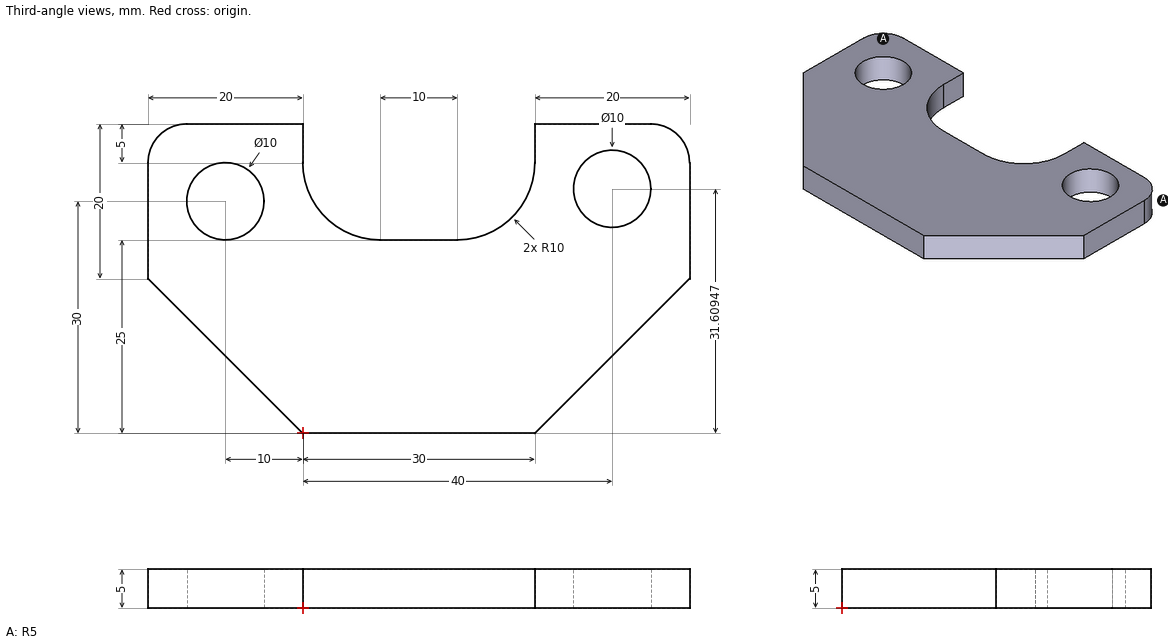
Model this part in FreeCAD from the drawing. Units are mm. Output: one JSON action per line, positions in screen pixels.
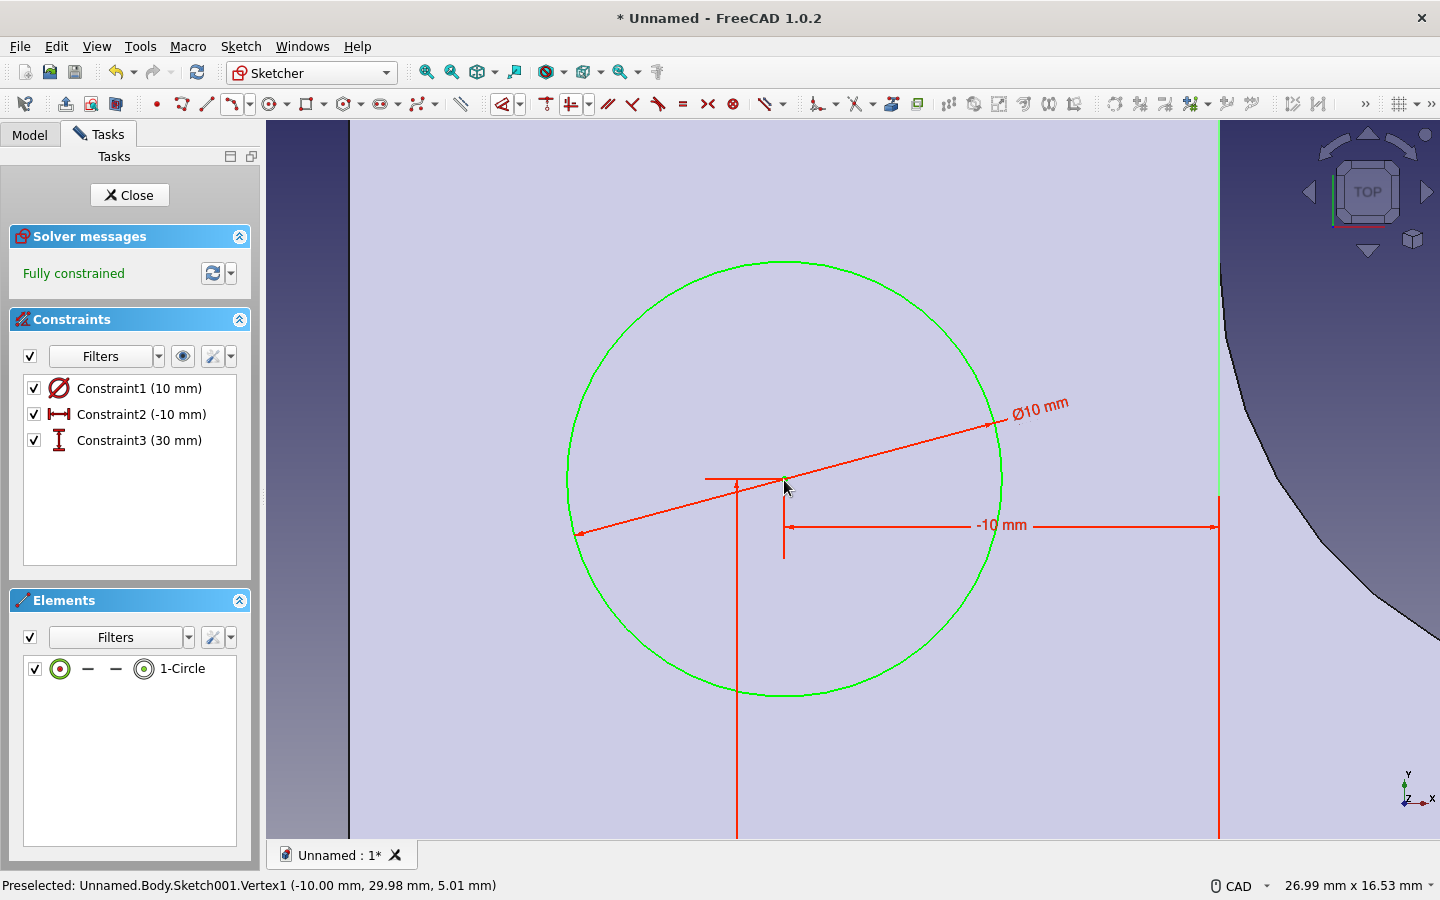
{"action": "left_click", "coordinate": [130, 195]}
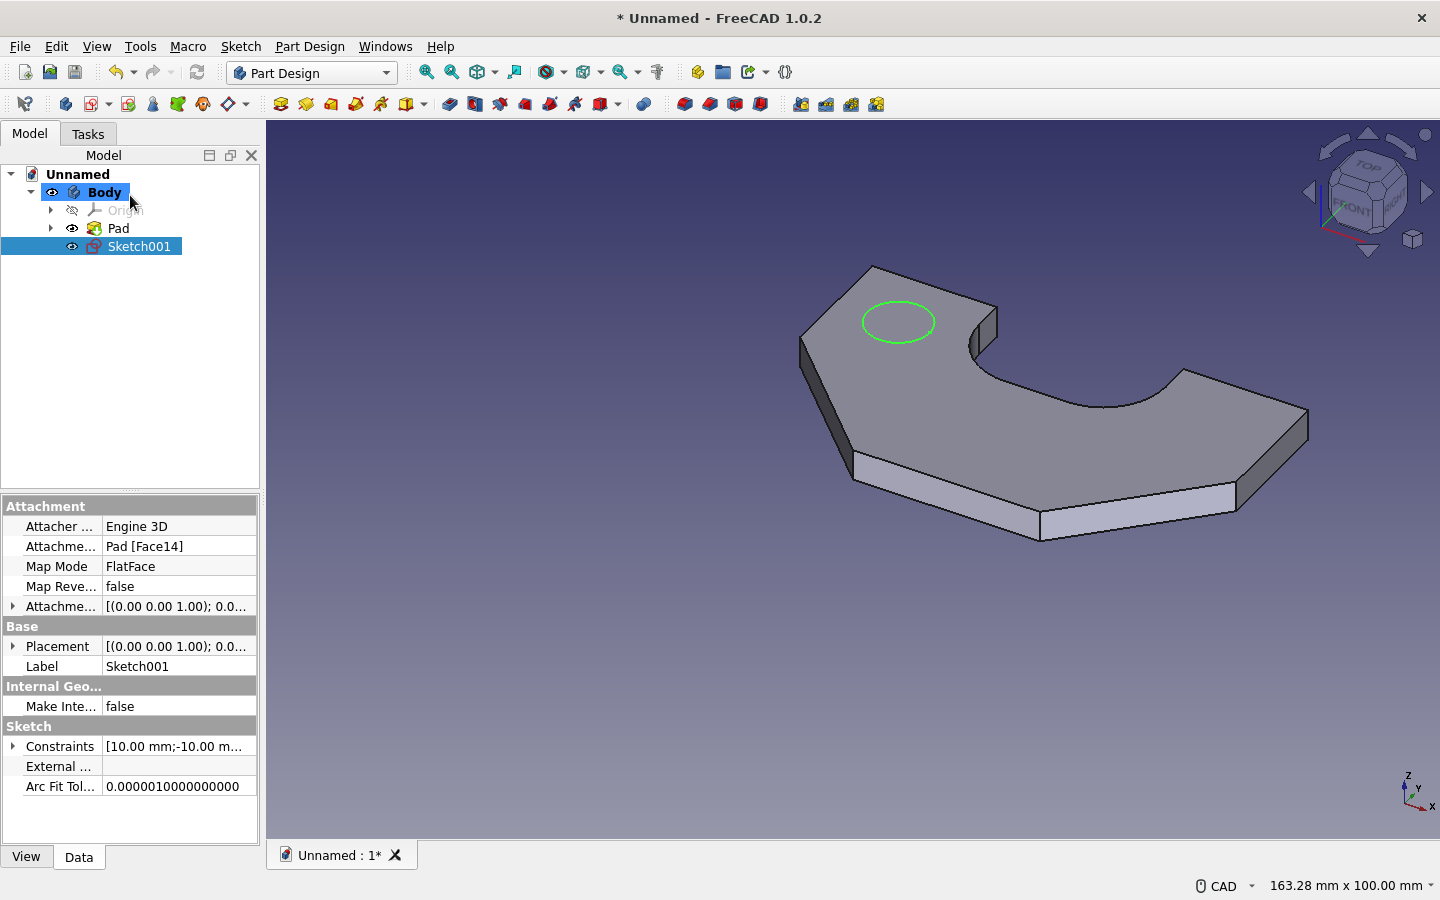
{"action": "left_click", "coordinate": [450, 104]}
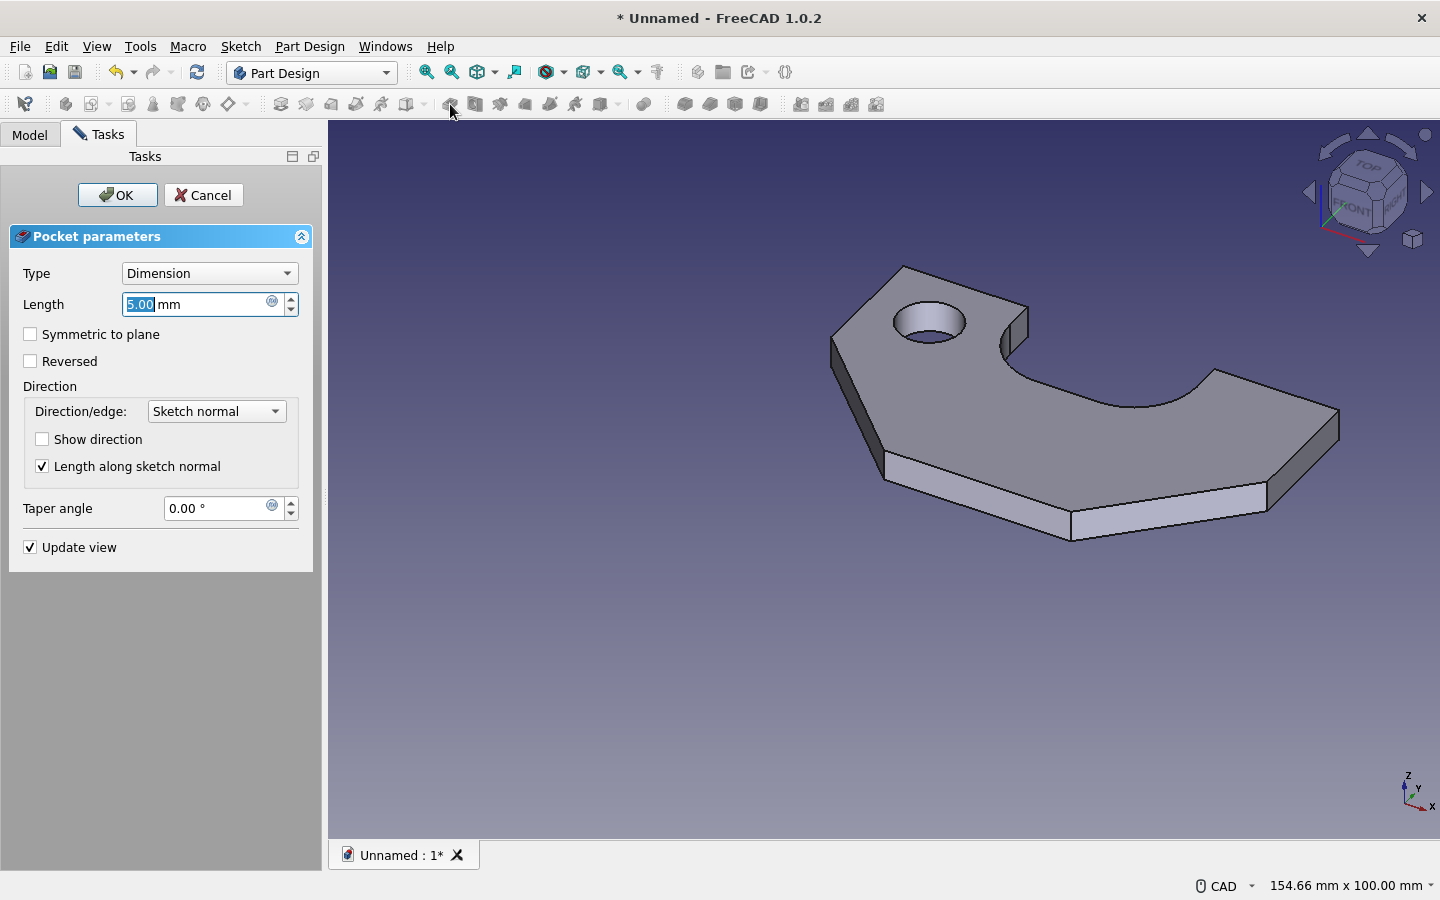
{"action": "type", "text": "5"}
{"action": "key", "text": "Tab"}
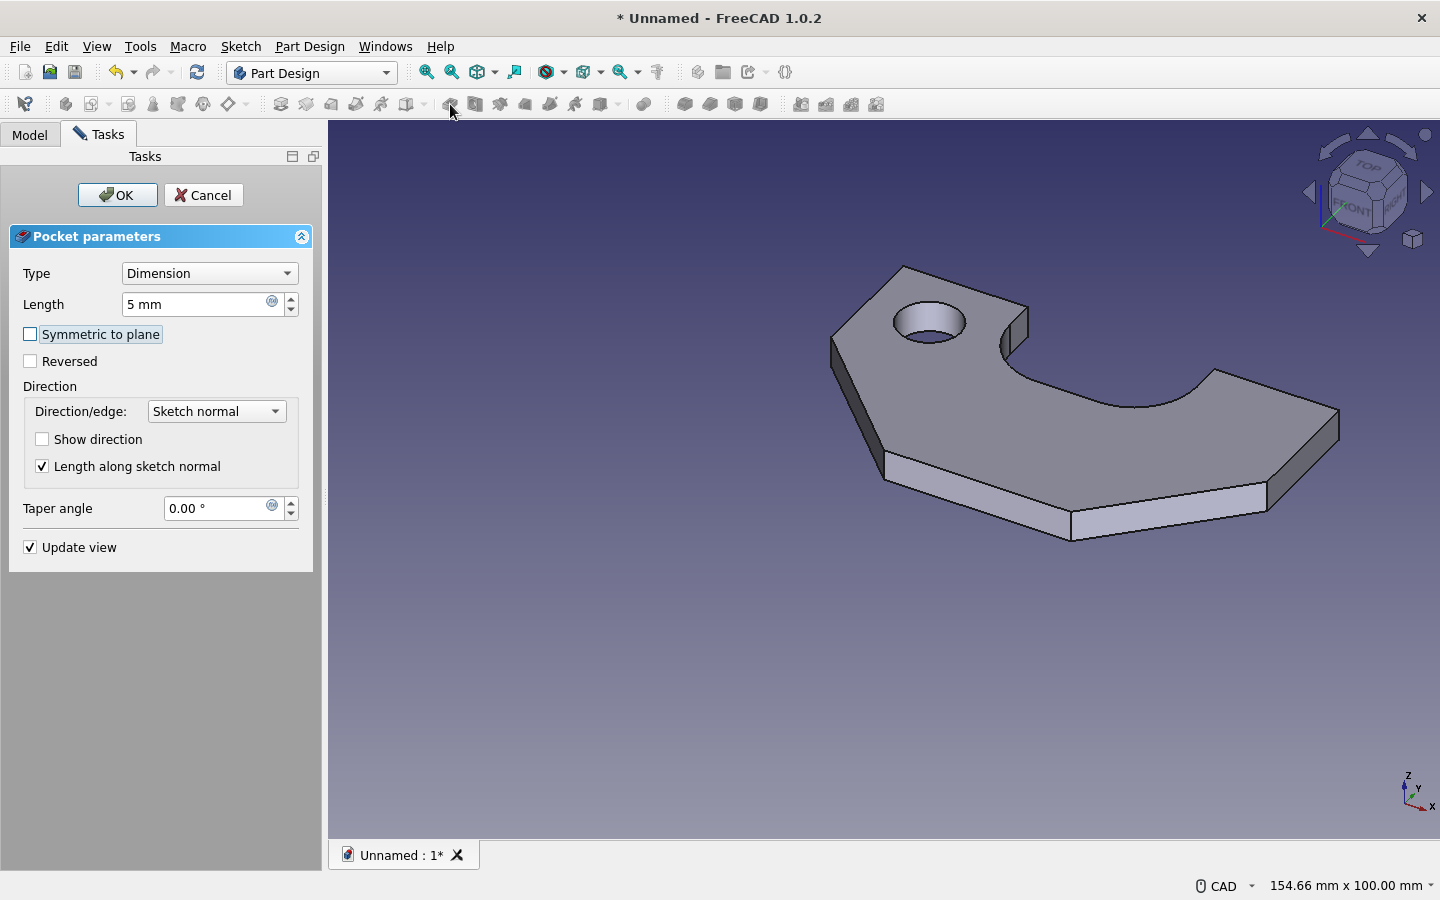
{"action": "left_click", "coordinate": [118, 195]}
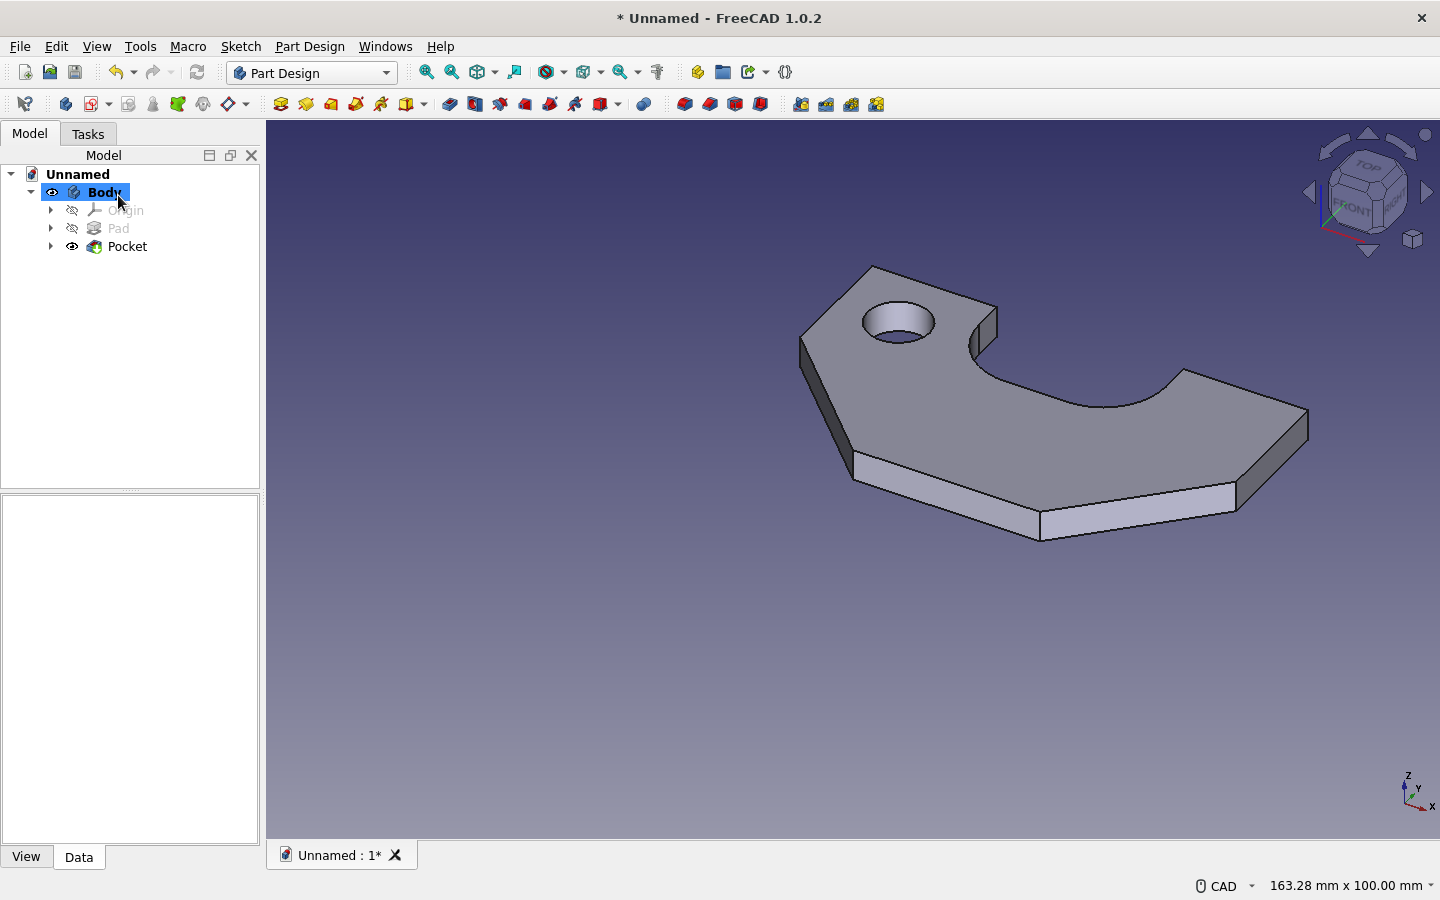
{"action": "left_click", "coordinate": [1060, 450]}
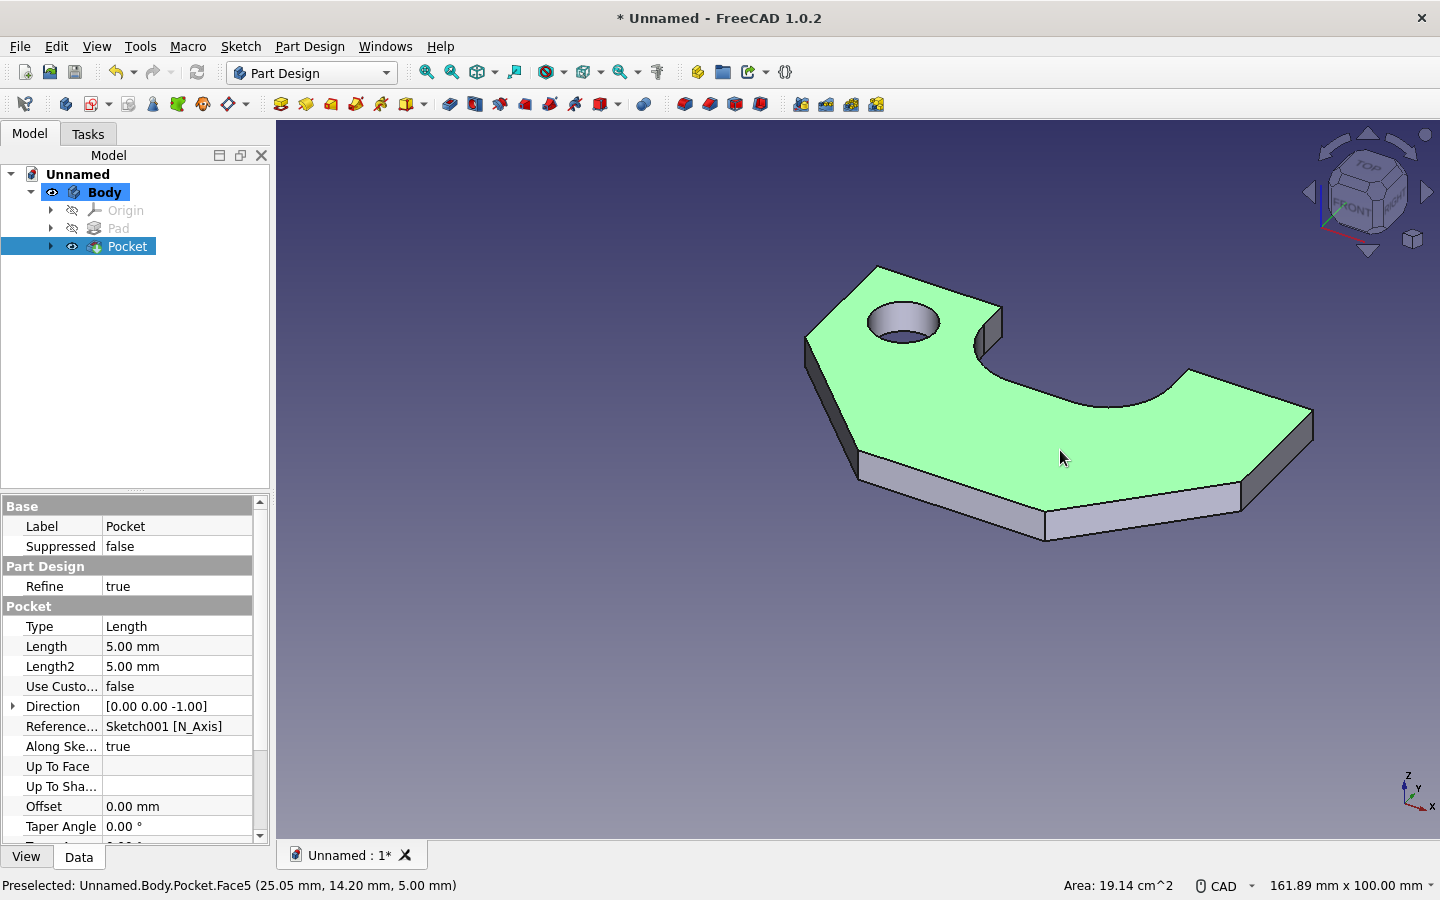
{"action": "left_click", "coordinate": [90, 104]}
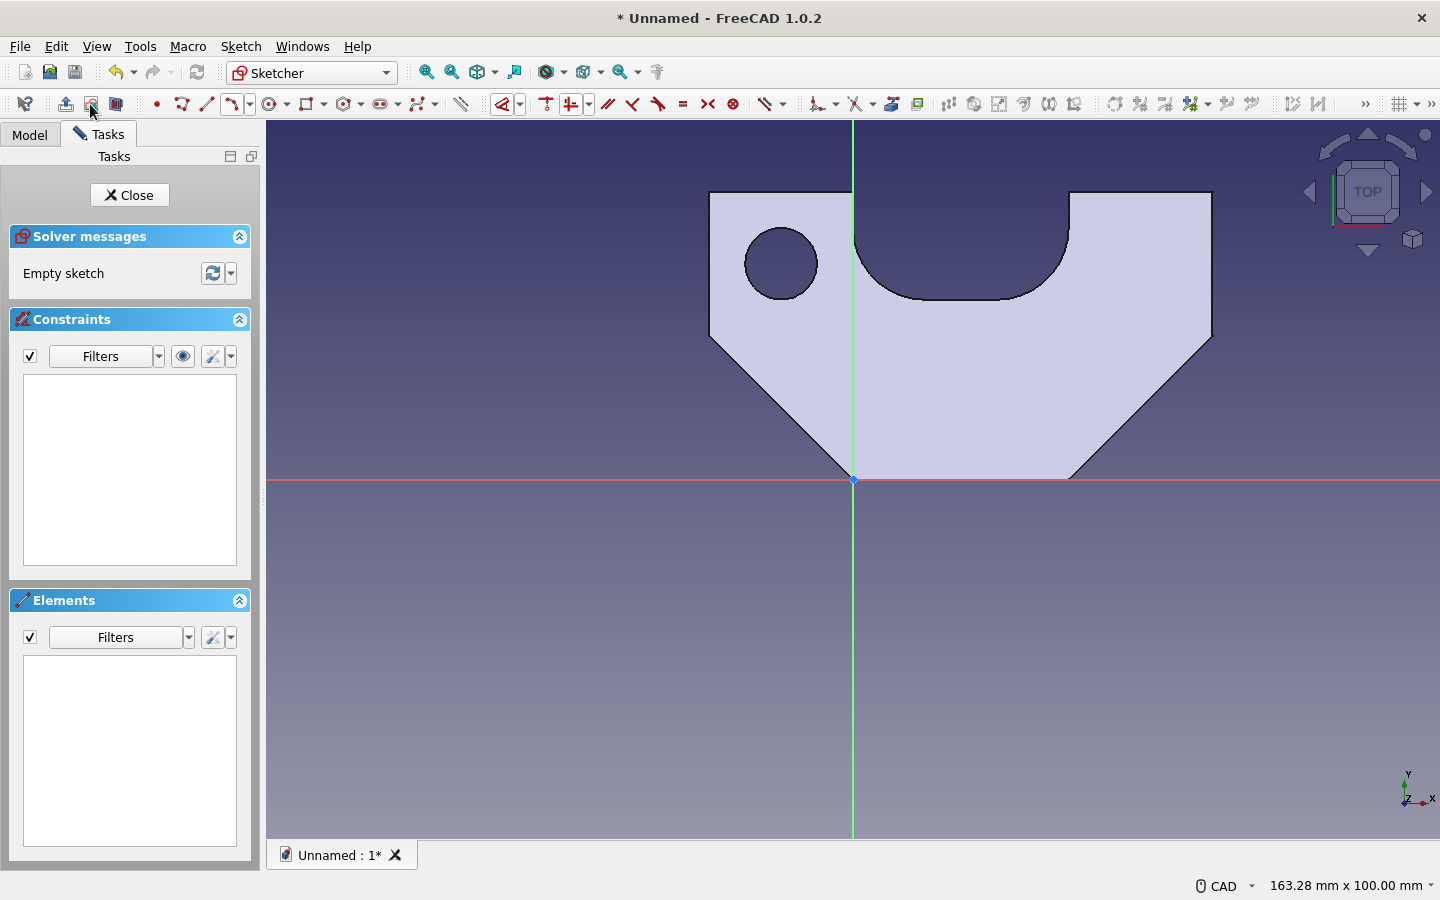
{"action": "scroll", "coordinate": [1211, 207], "scroll_direction": "up", "scroll_amount": 9}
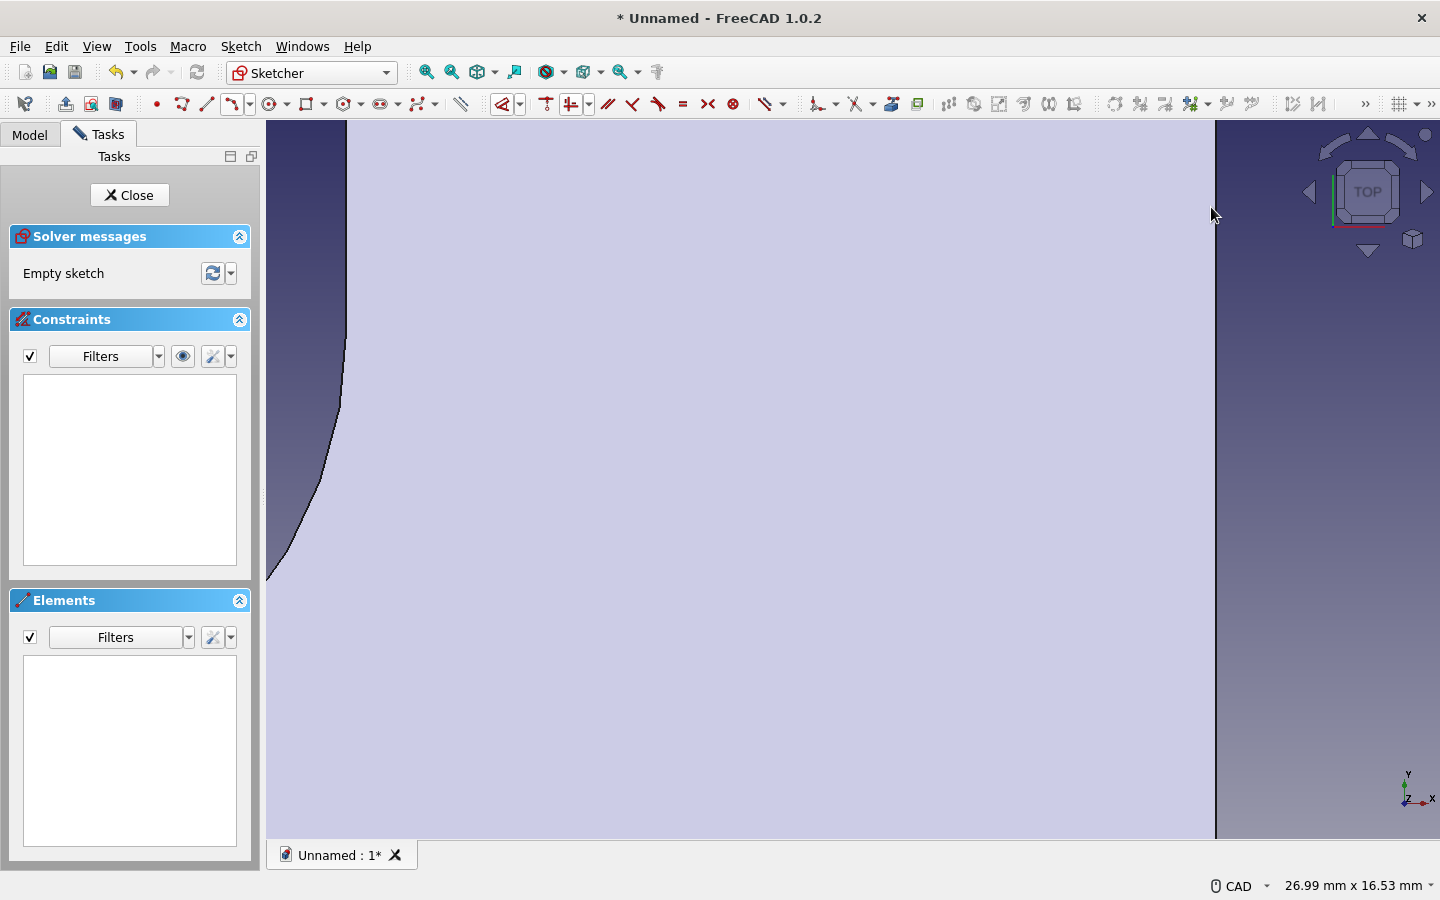
{"action": "left_click", "coordinate": [268, 104]}